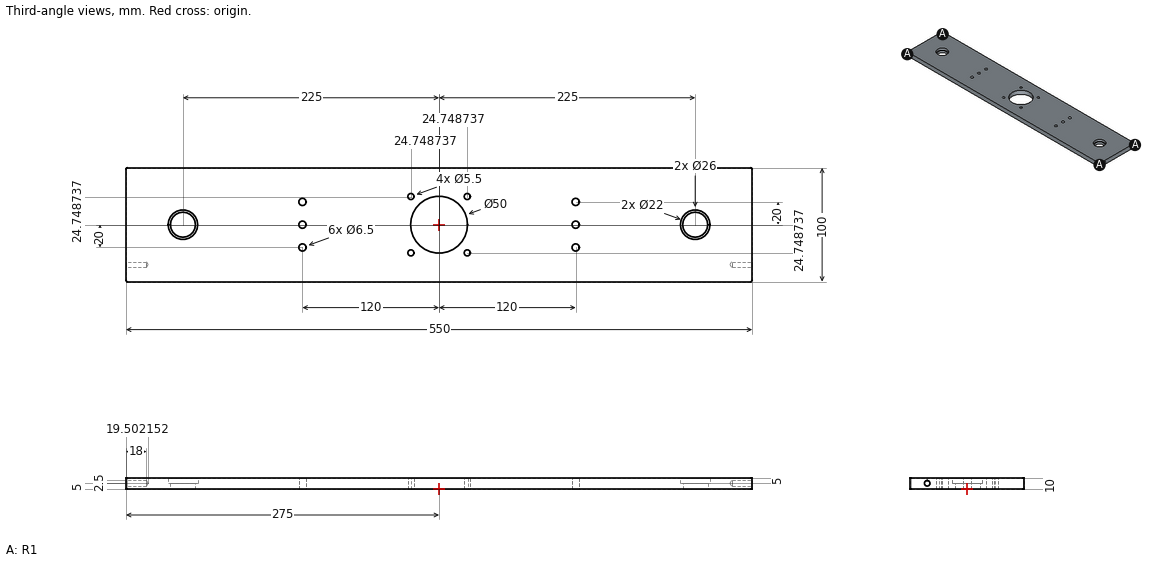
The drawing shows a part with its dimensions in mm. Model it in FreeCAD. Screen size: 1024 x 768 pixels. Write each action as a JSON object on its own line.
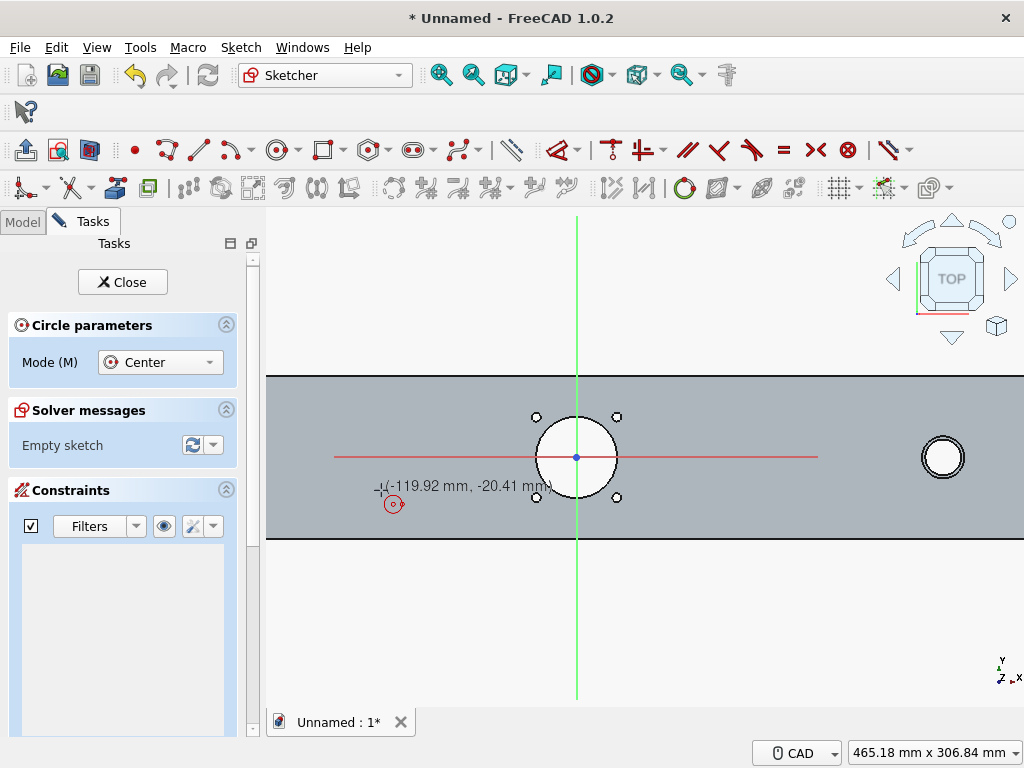
{"action": "left_click", "coordinate": [381, 490]}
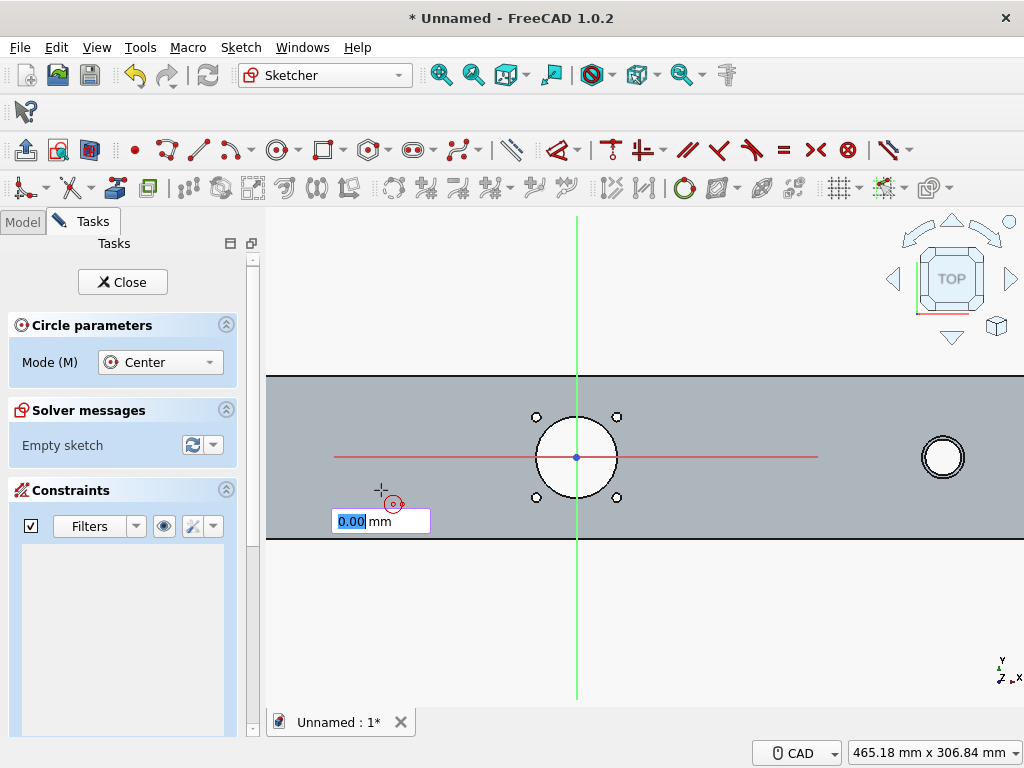
{"action": "scroll", "coordinate": [385, 486], "scroll_direction": "up", "scroll_amount": 6}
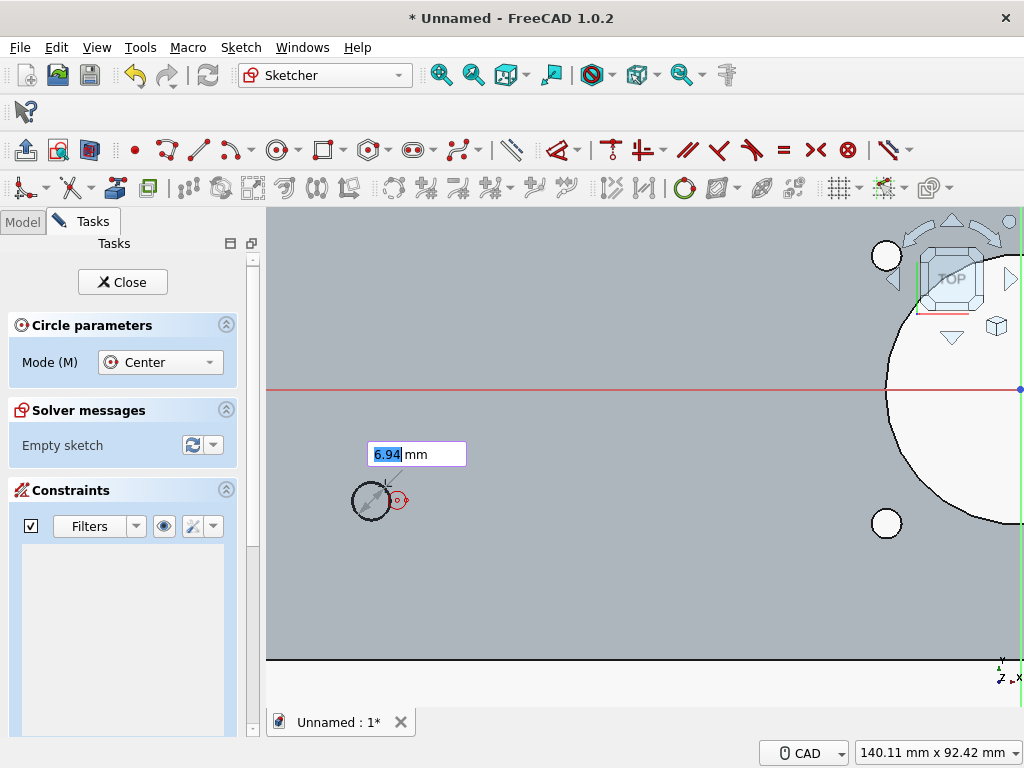
{"action": "left_click", "coordinate": [384, 485]}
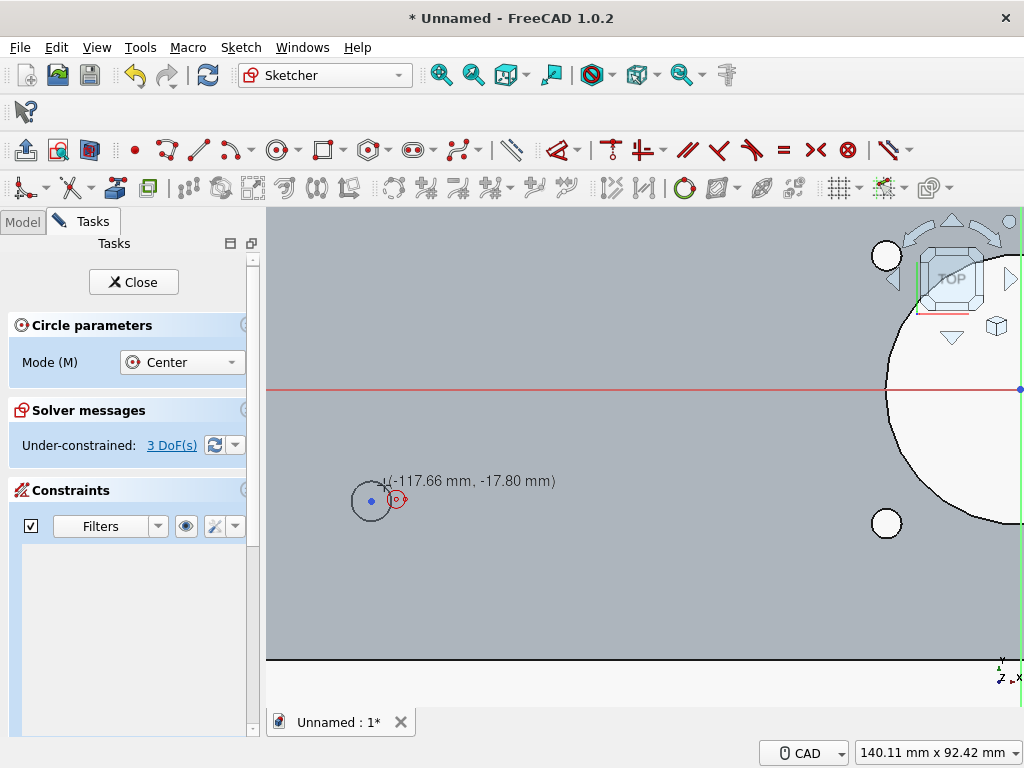
{"action": "scroll", "coordinate": [385, 486], "scroll_direction": "down", "scroll_amount": 6}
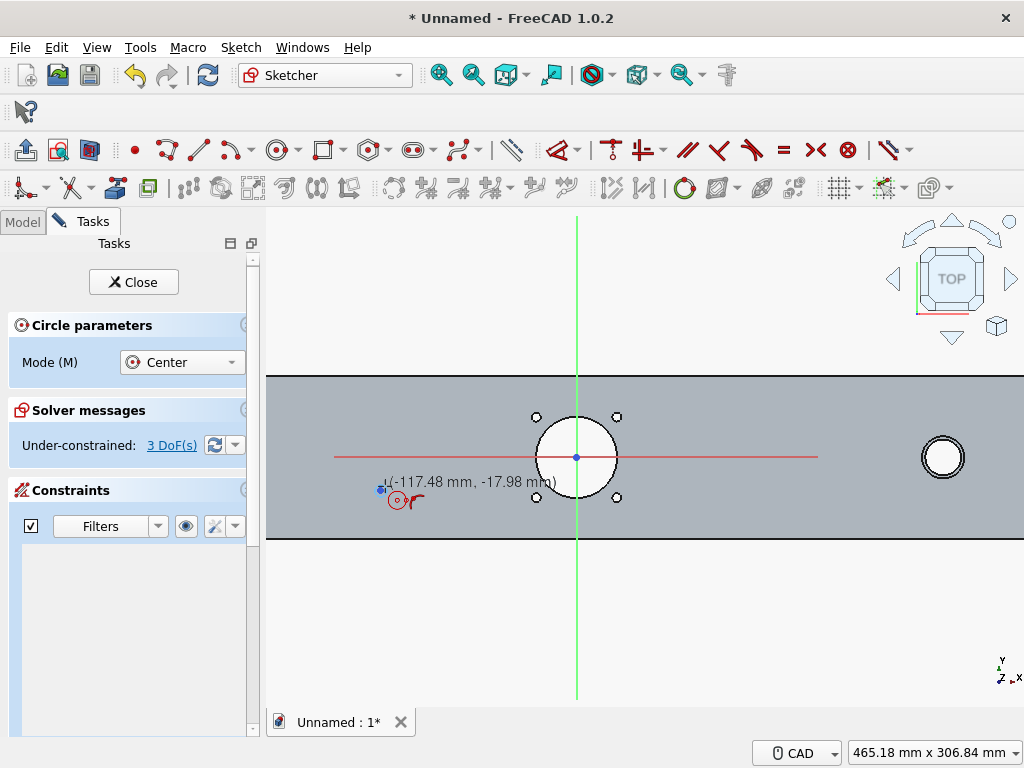
{"action": "scroll", "coordinate": [772, 490], "scroll_direction": "up", "scroll_amount": 8}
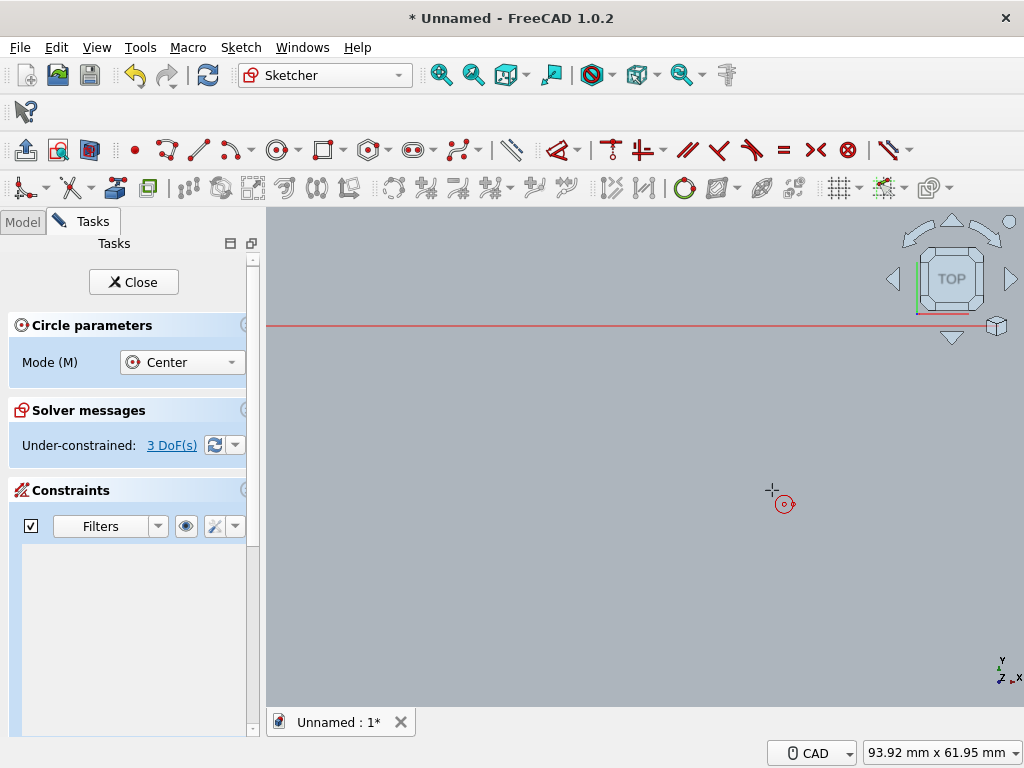
{"action": "scroll", "coordinate": [773, 490], "scroll_direction": "down", "scroll_amount": 8}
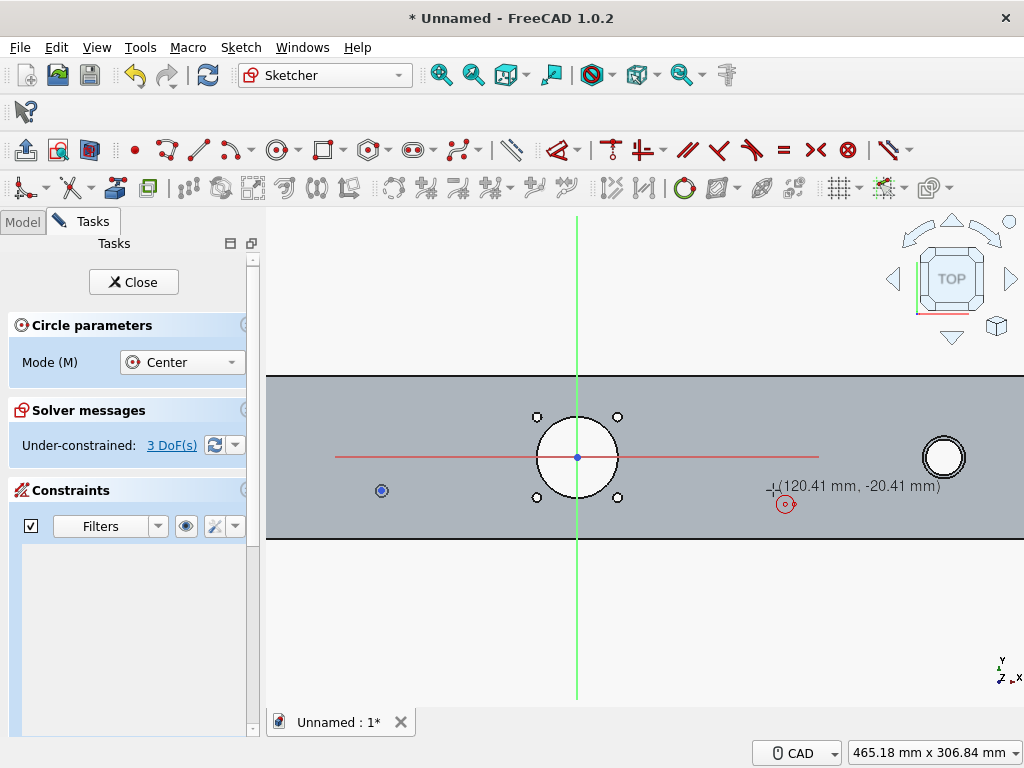
{"action": "left_click", "coordinate": [773, 490]}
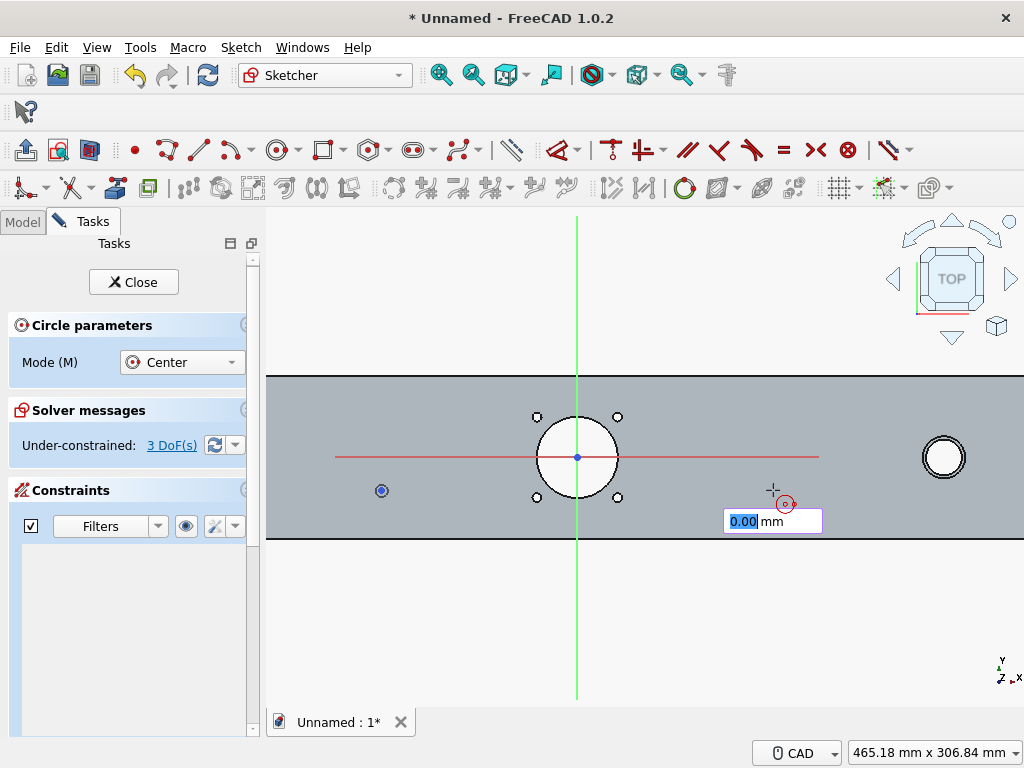
{"action": "scroll", "coordinate": [777, 486], "scroll_direction": "up", "scroll_amount": 6}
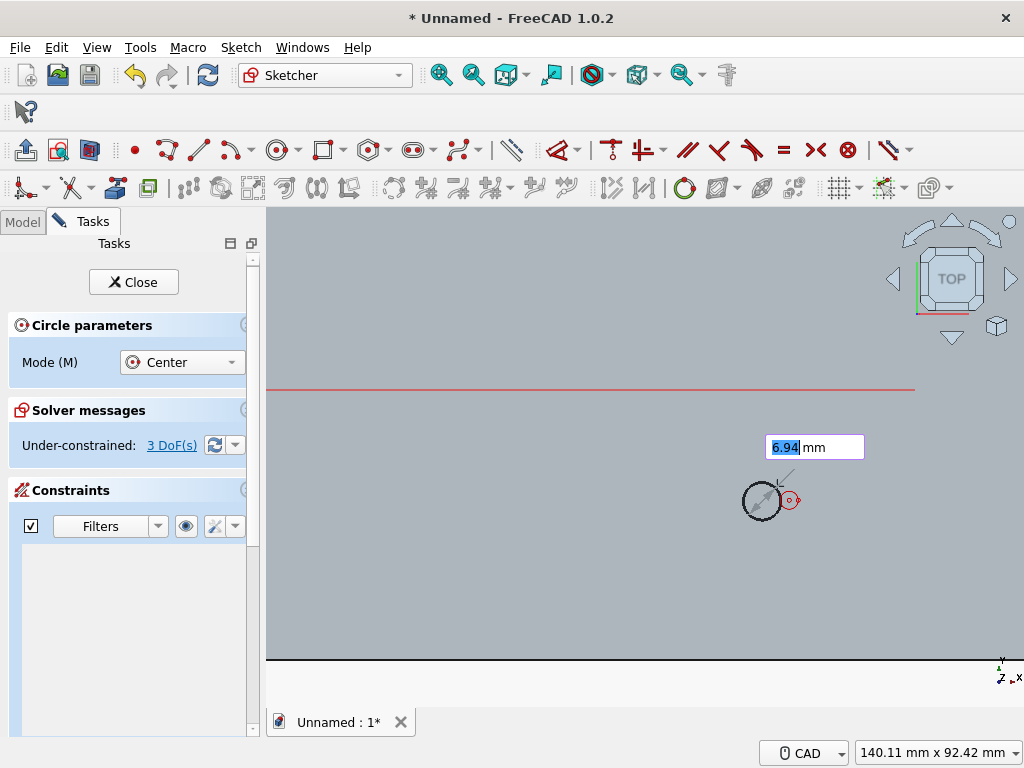
{"action": "left_click", "coordinate": [774, 485]}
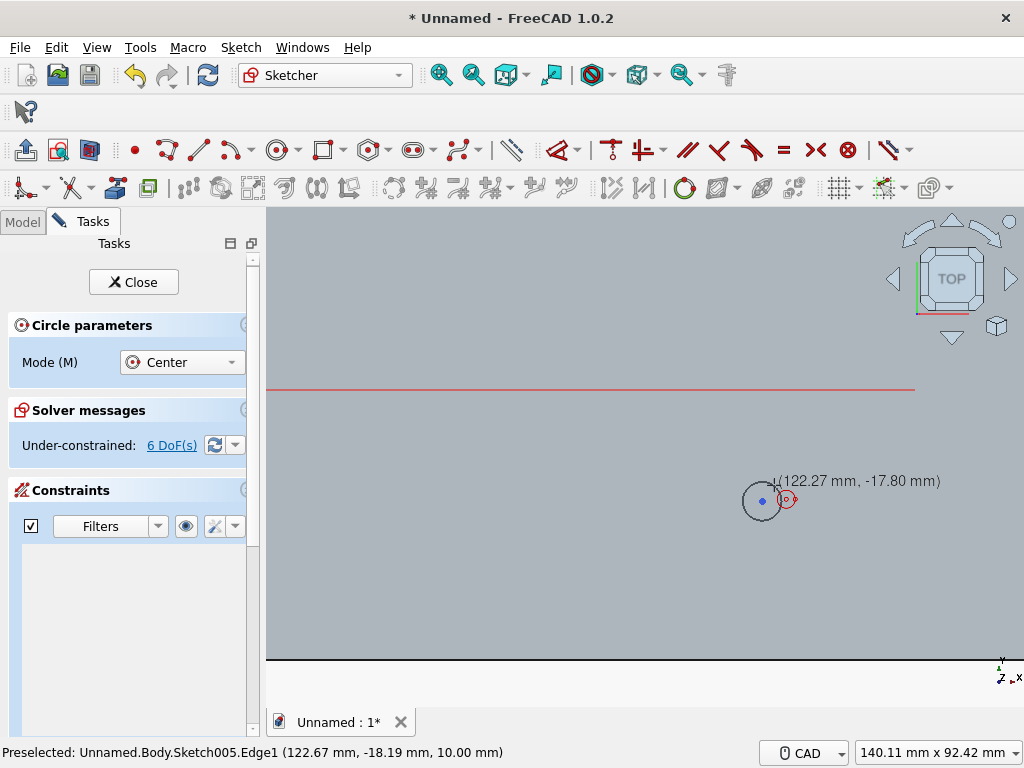
{"action": "scroll", "coordinate": [762, 282], "scroll_direction": "up", "scroll_amount": 2}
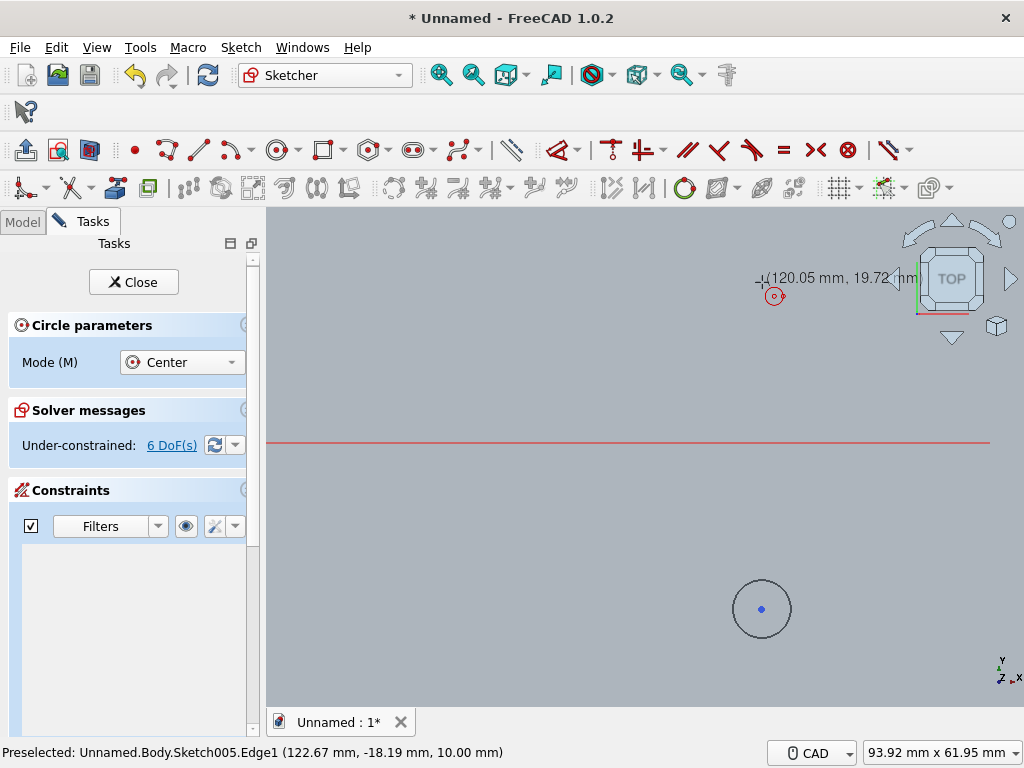
{"action": "scroll", "coordinate": [775, 461], "scroll_direction": "down", "scroll_amount": 8}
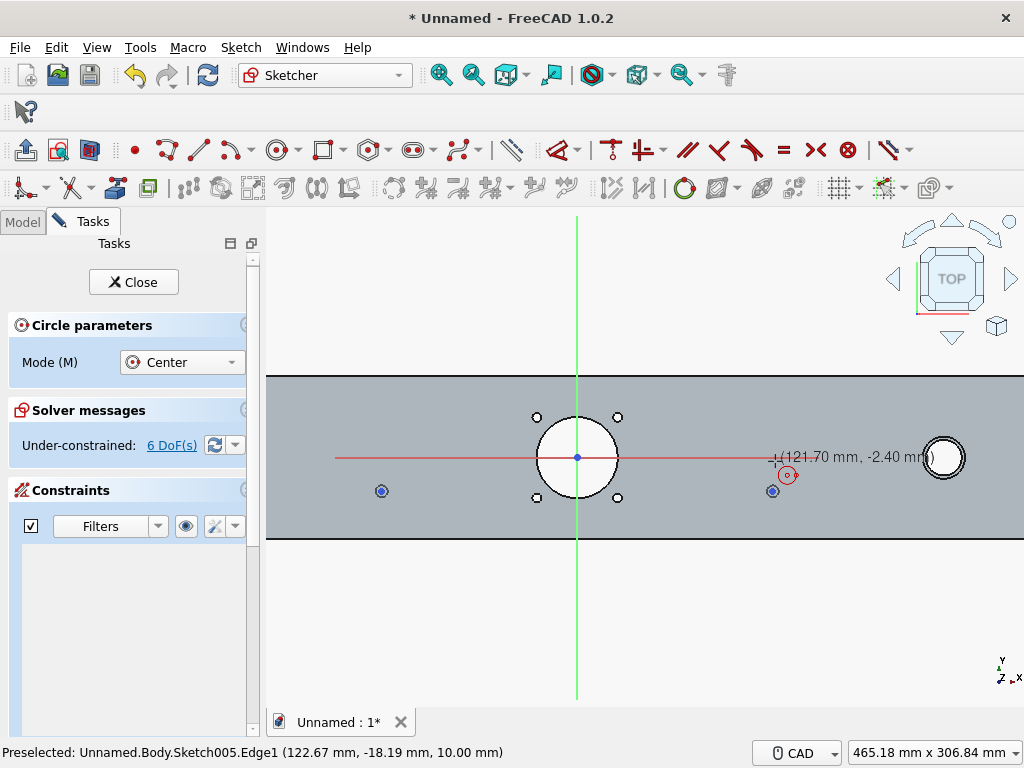
{"action": "left_click", "coordinate": [773, 425]}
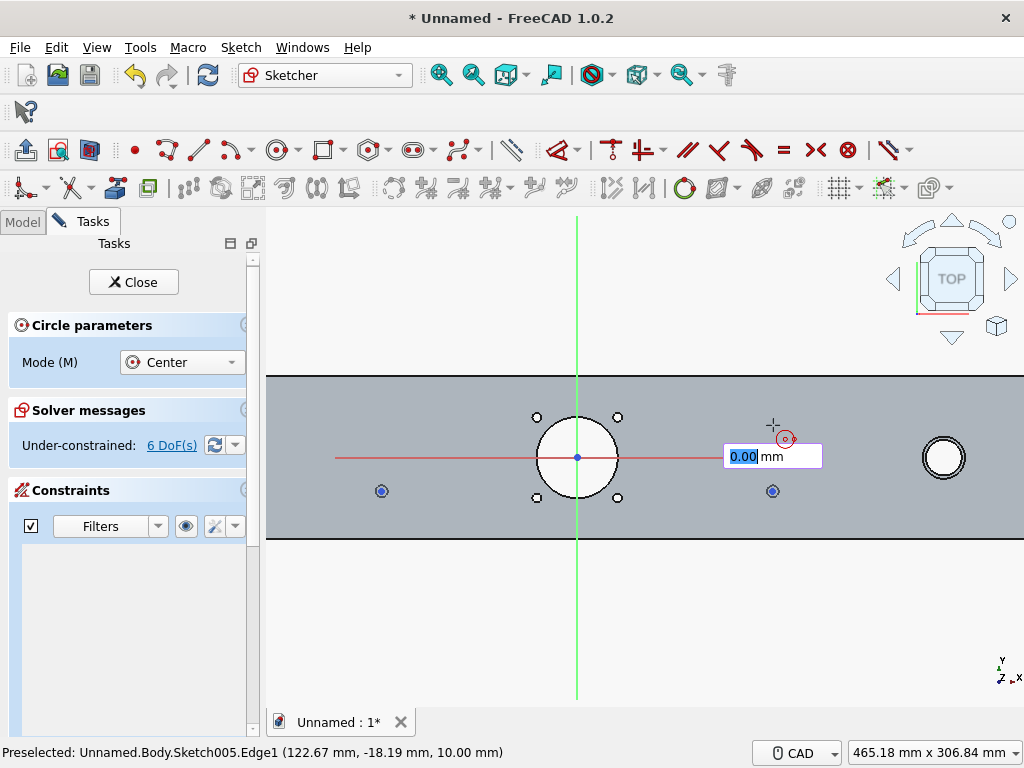
{"action": "scroll", "coordinate": [777, 421], "scroll_direction": "up", "scroll_amount": 6}